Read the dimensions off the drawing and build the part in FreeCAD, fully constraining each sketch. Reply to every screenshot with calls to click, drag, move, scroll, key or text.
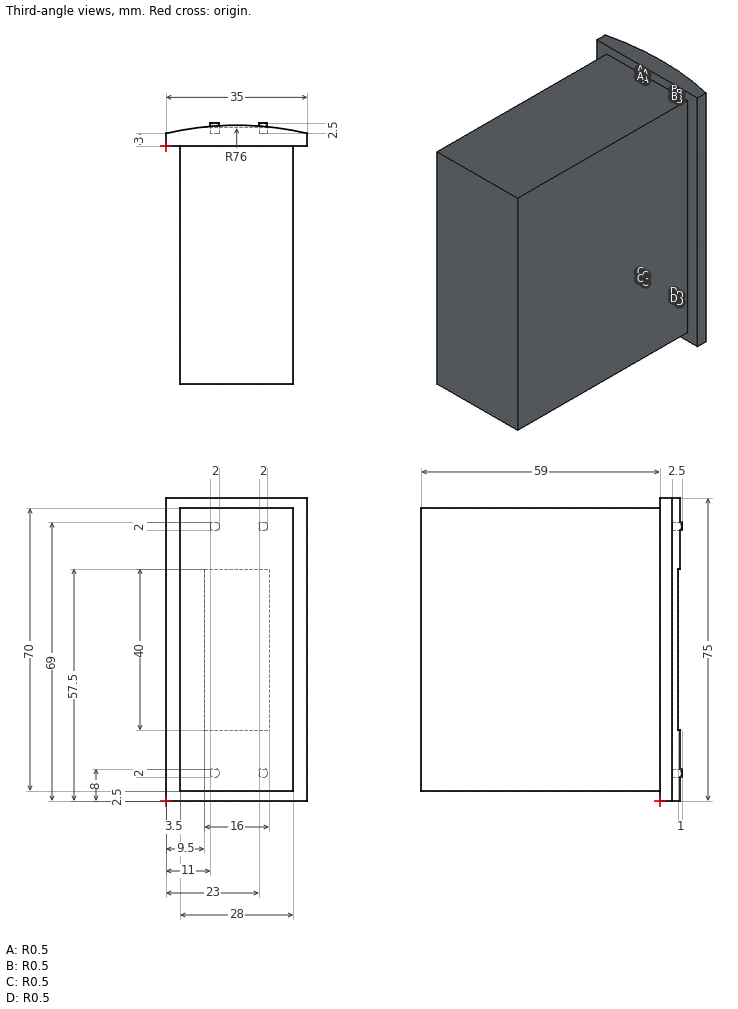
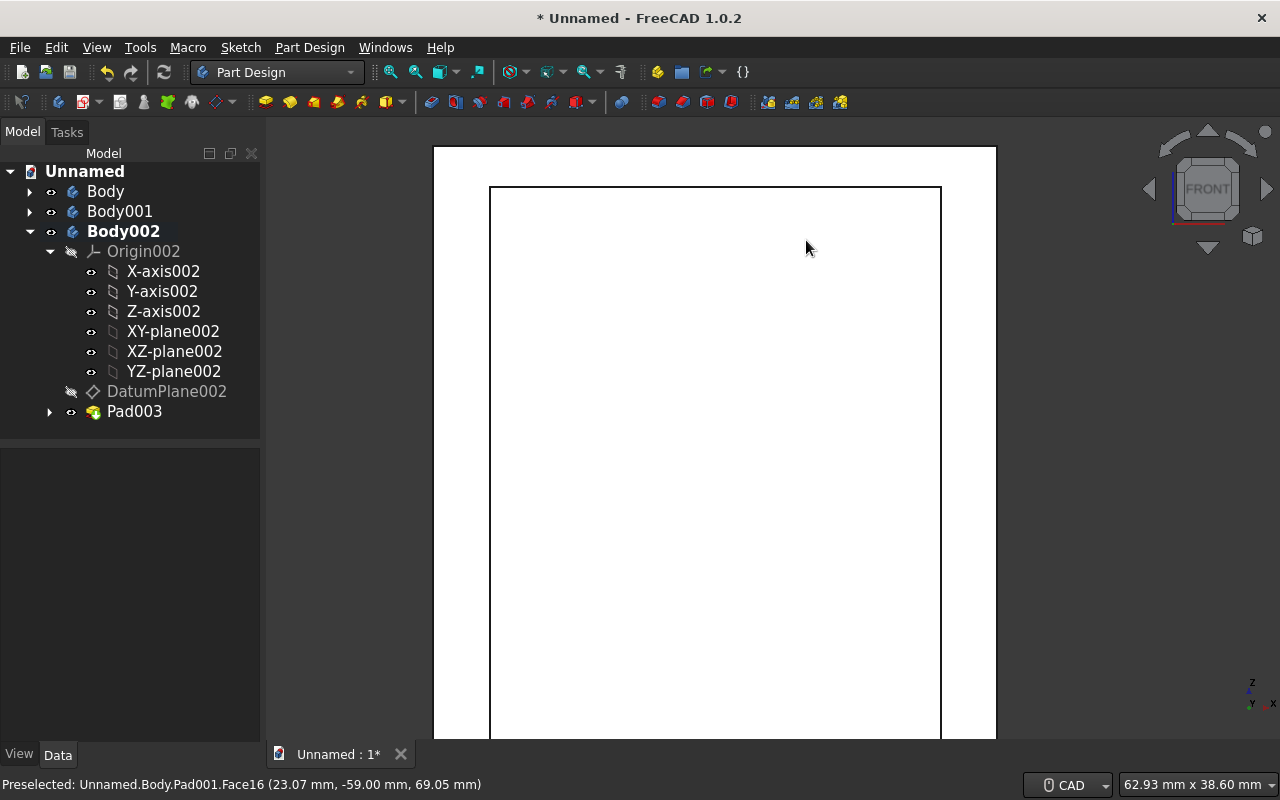
click(392, 72)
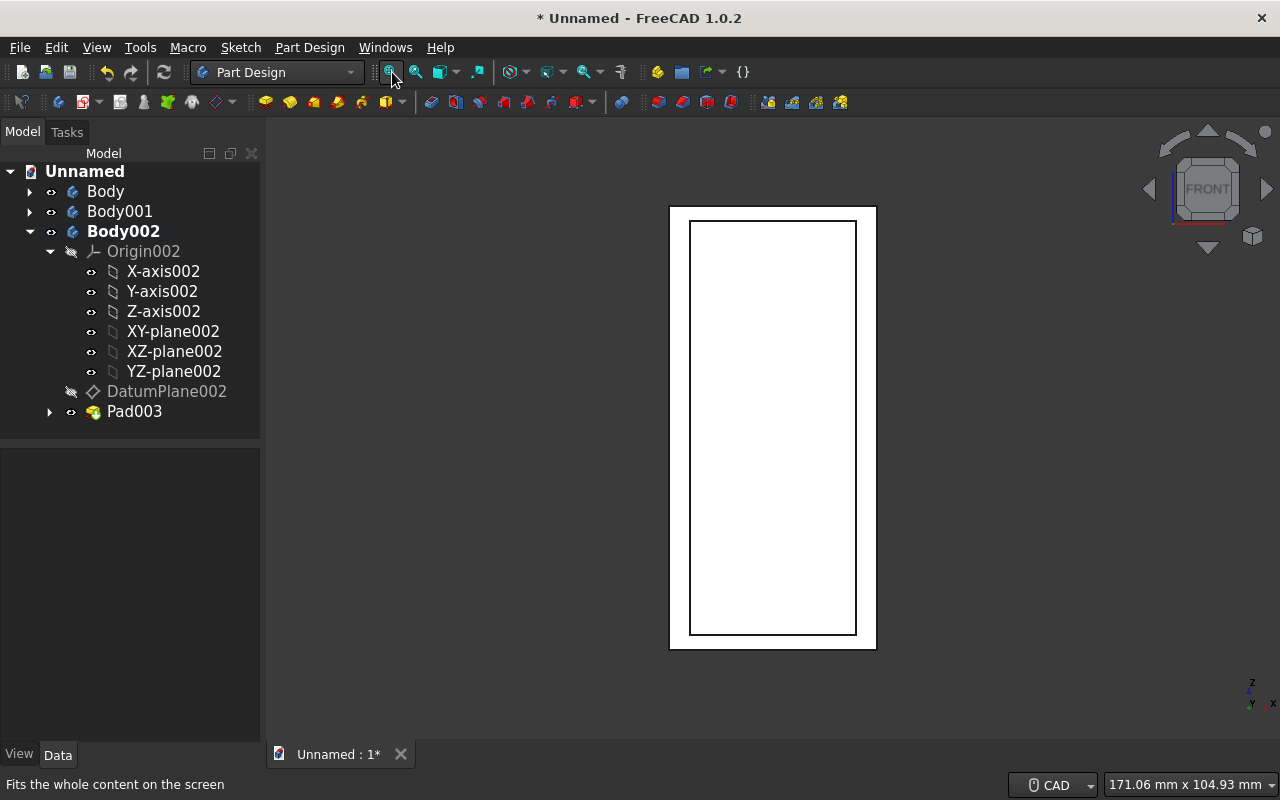
key(3)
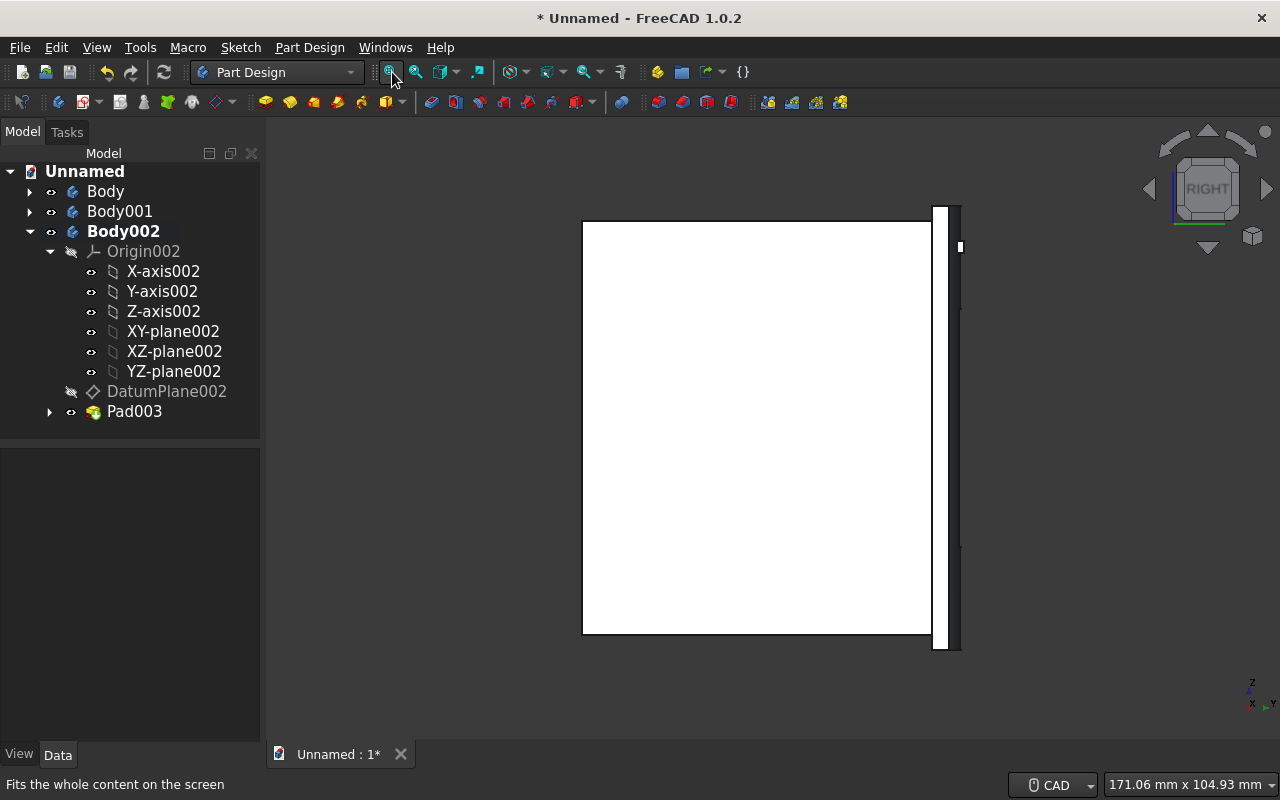
key(v)
key(f)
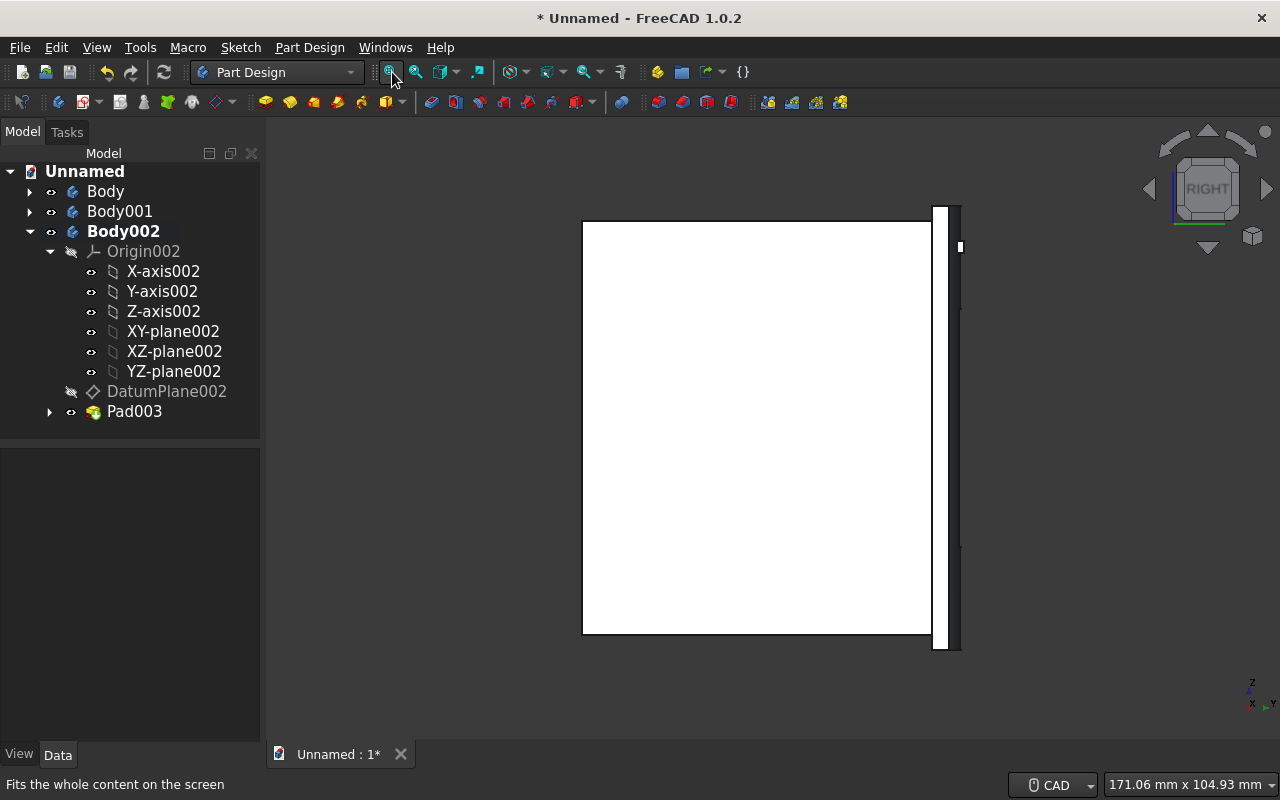
scroll(957, 240, up, 5)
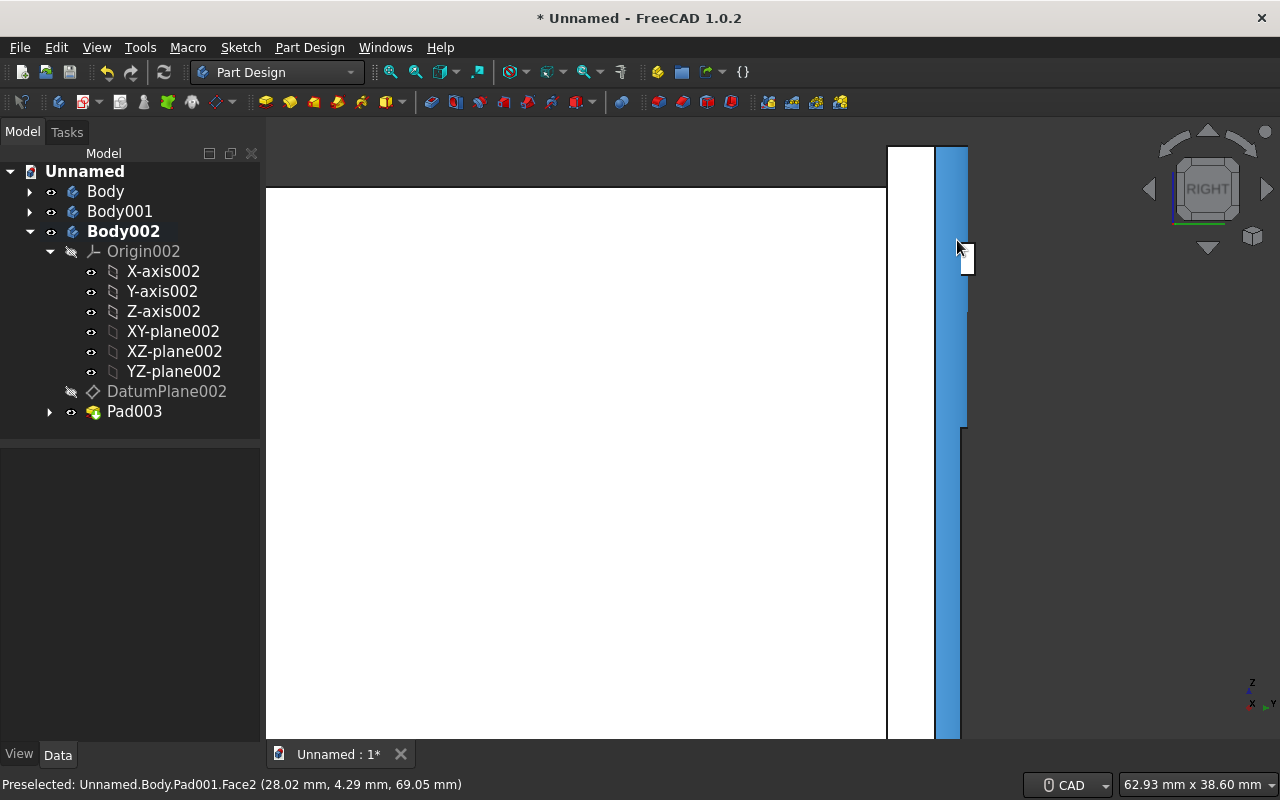
click(963, 242)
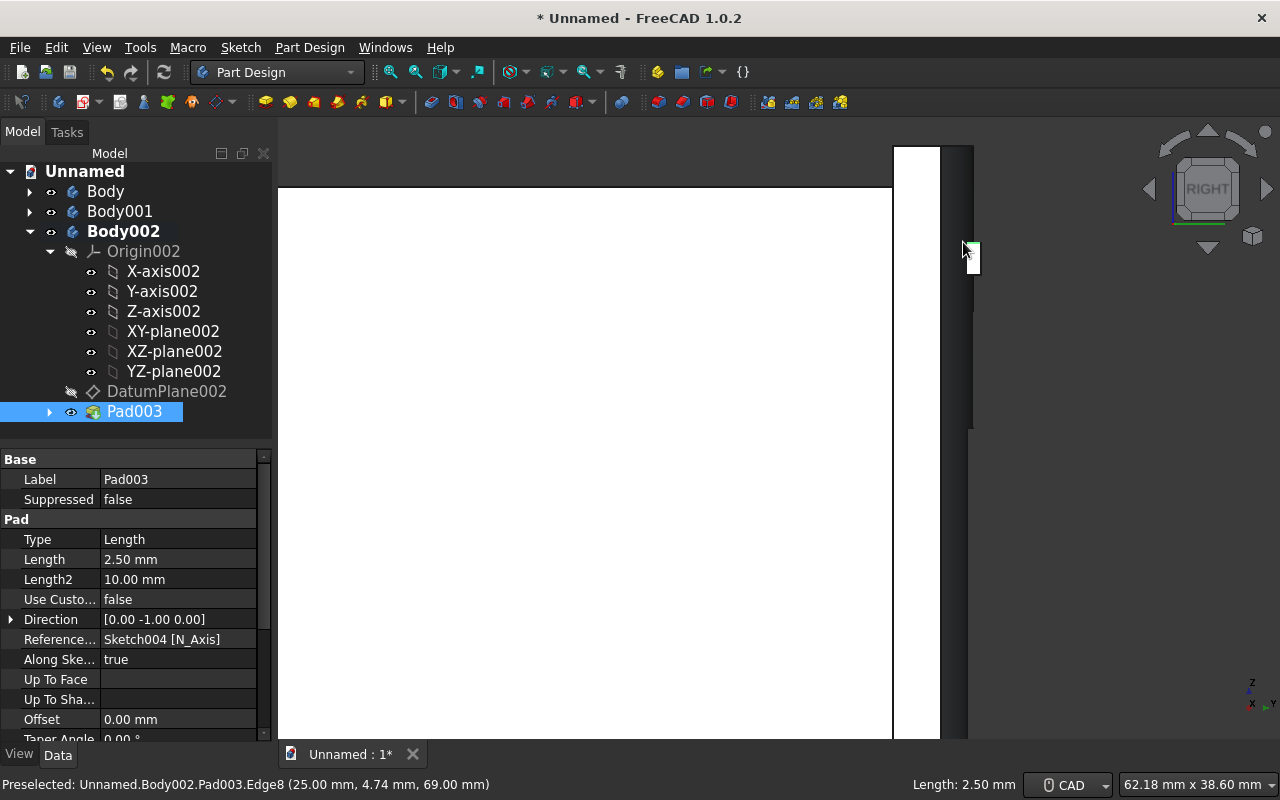
key(v)
key(f)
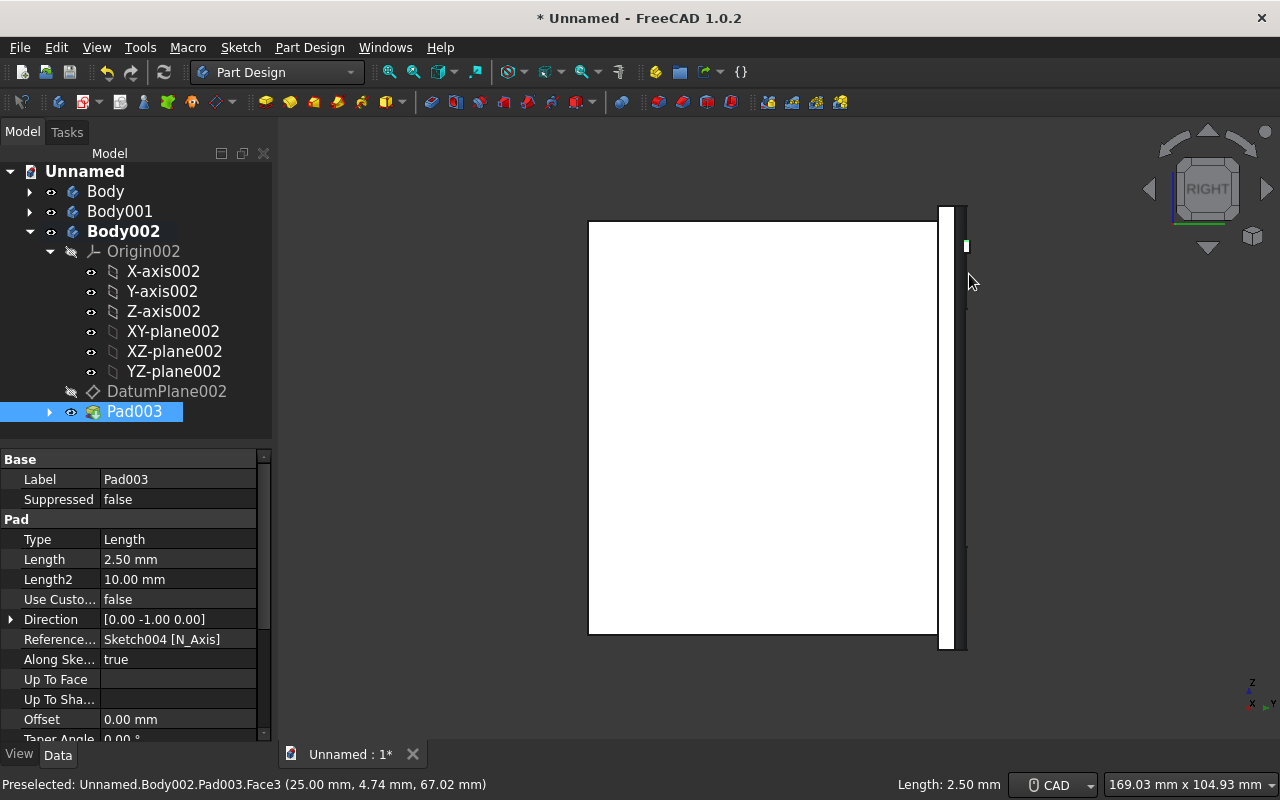
key(5)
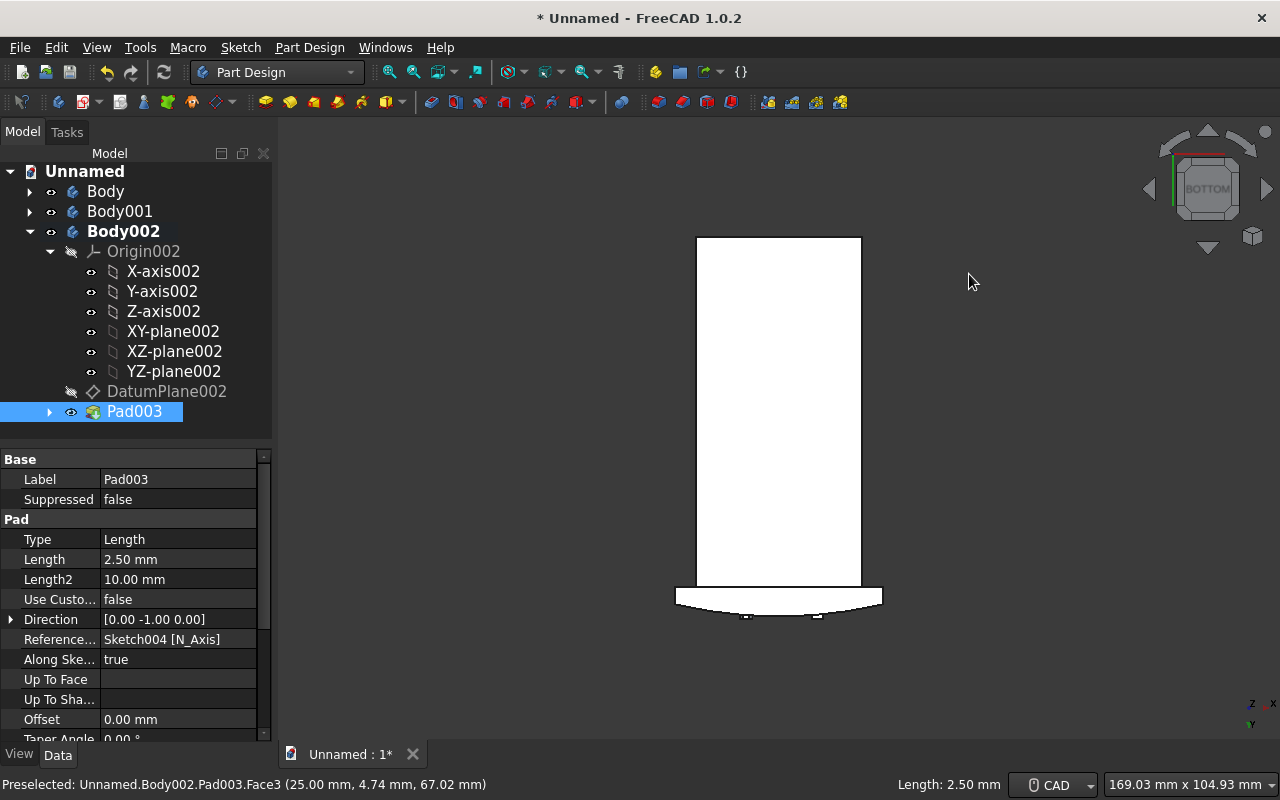
key(v)
key(f)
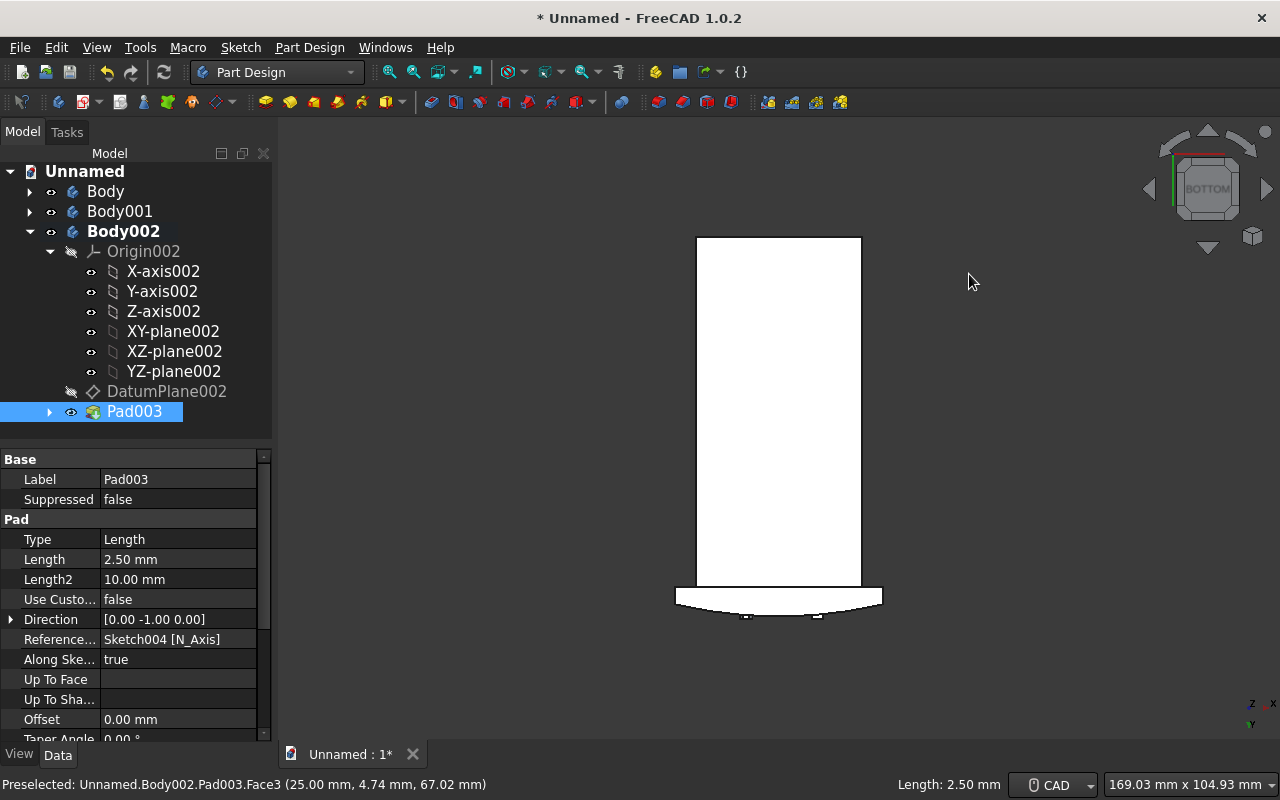
scroll(812, 611, up, 5)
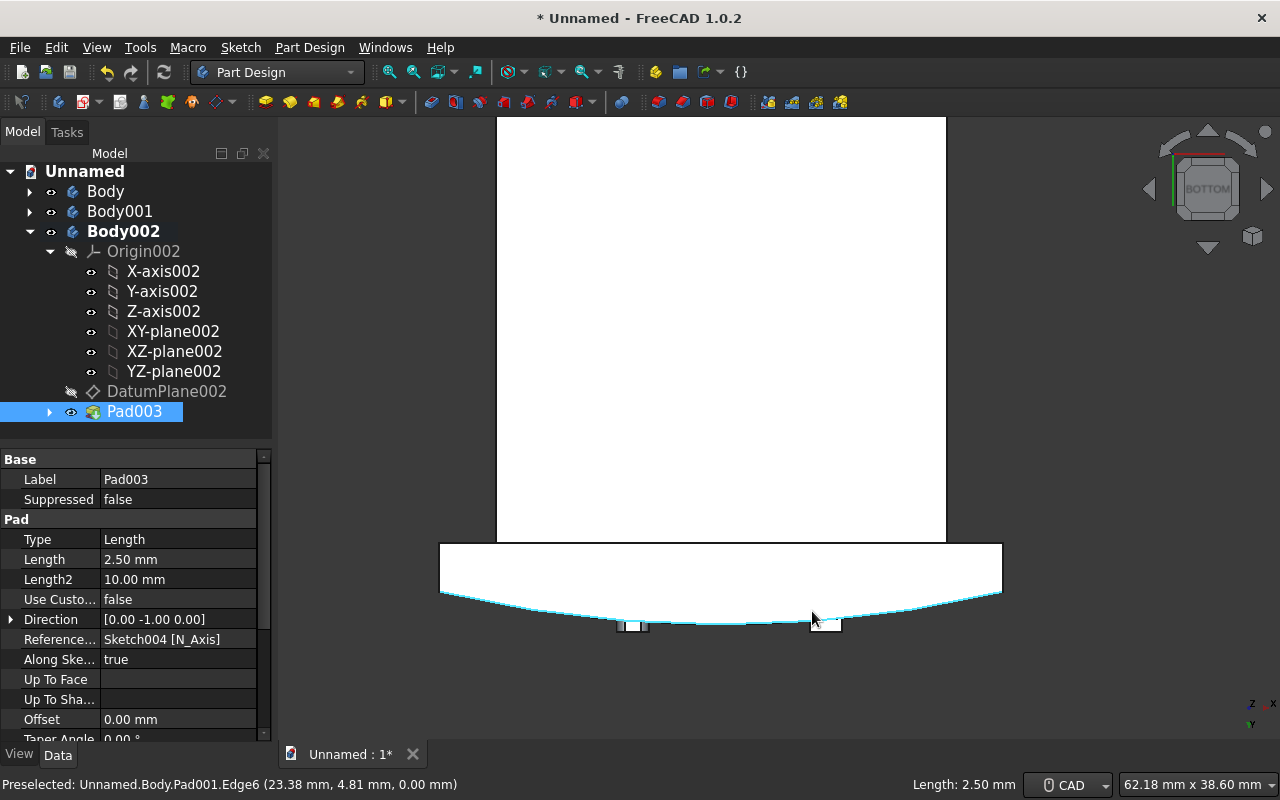
key(v)
key(f)